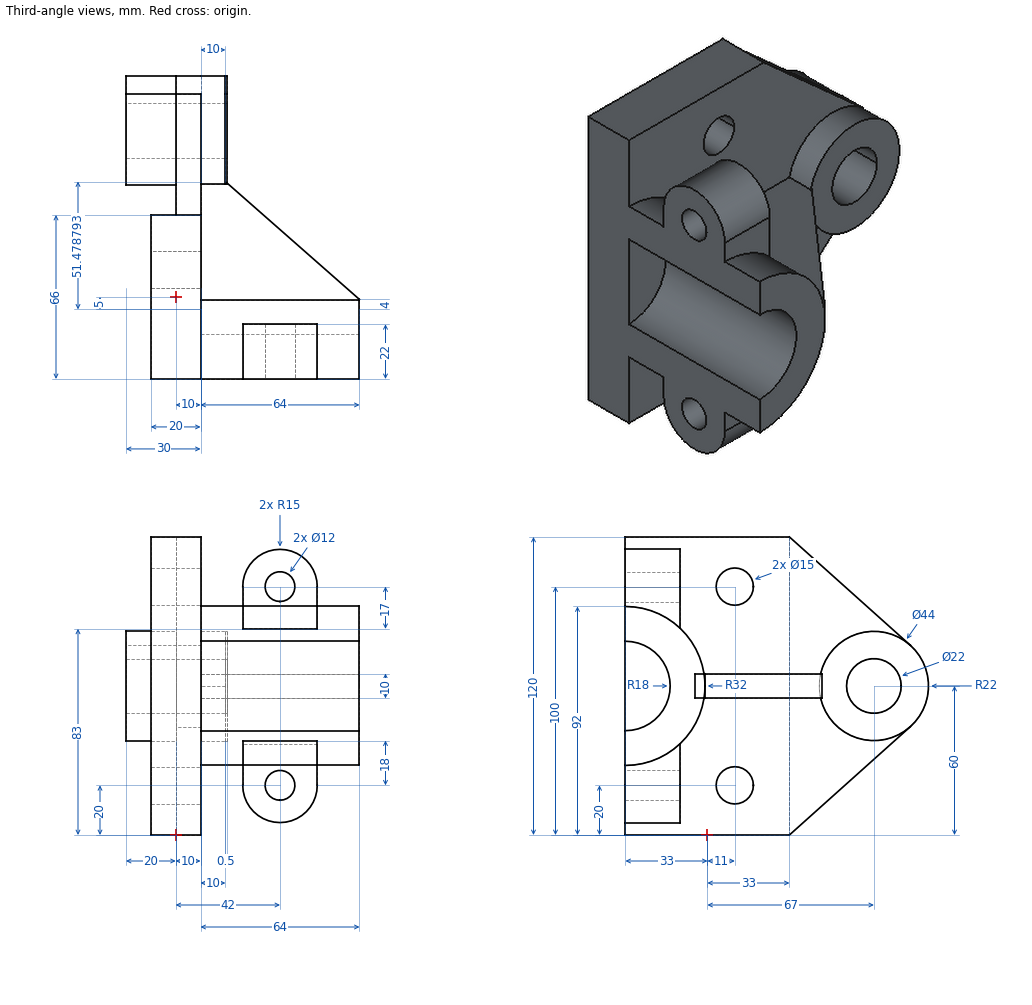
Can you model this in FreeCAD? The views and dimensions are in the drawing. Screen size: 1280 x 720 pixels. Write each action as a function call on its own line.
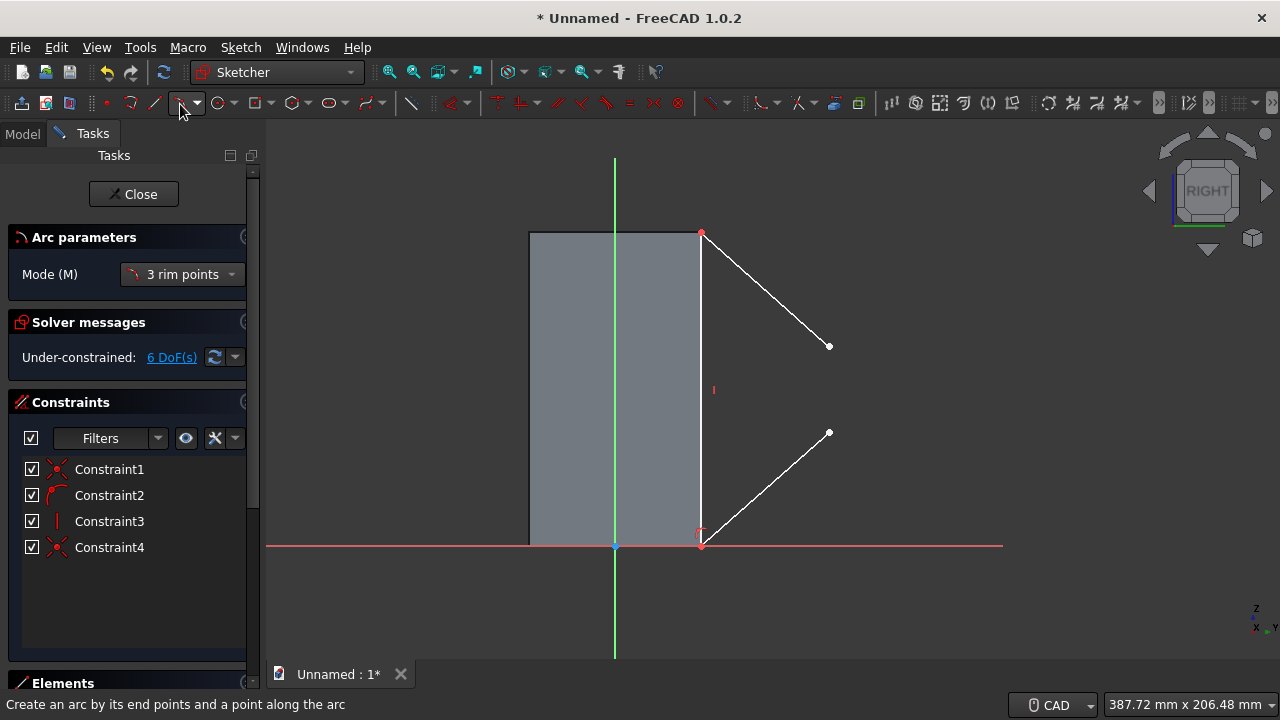
click(829, 433)
click(829, 347)
click(848, 389)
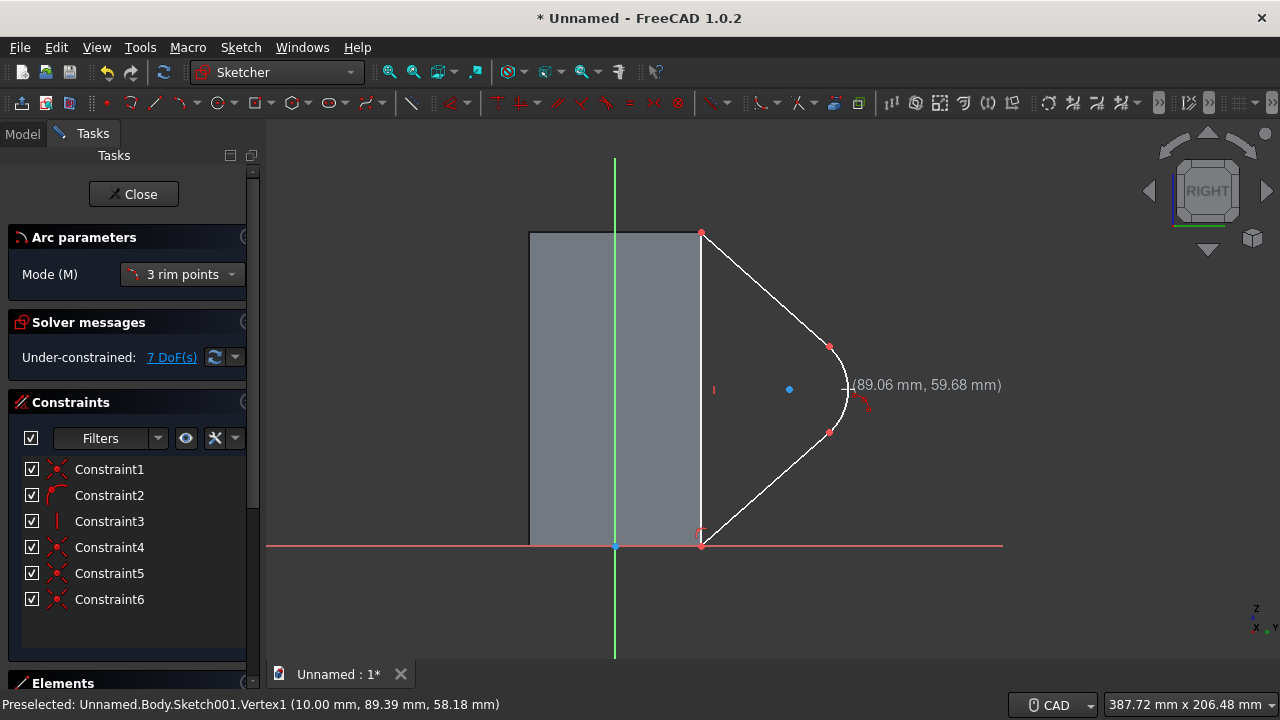
click(218, 104)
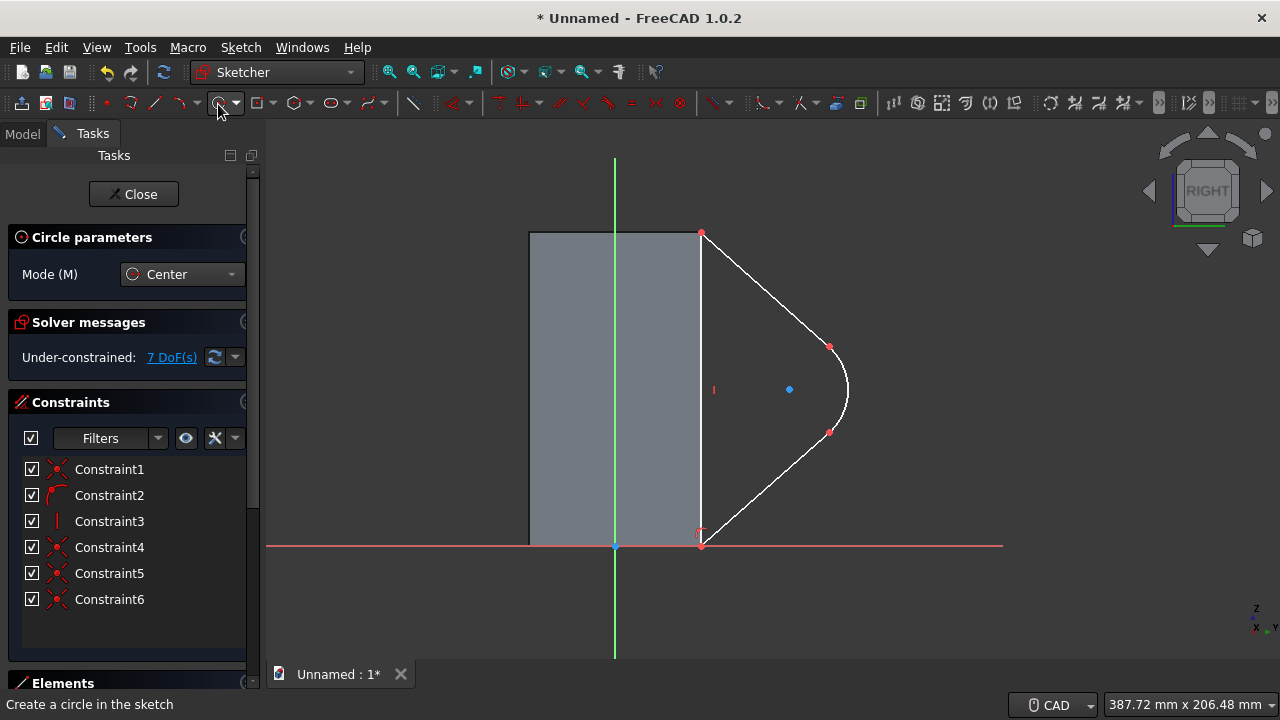
click(790, 389)
click(811, 369)
key(Escape)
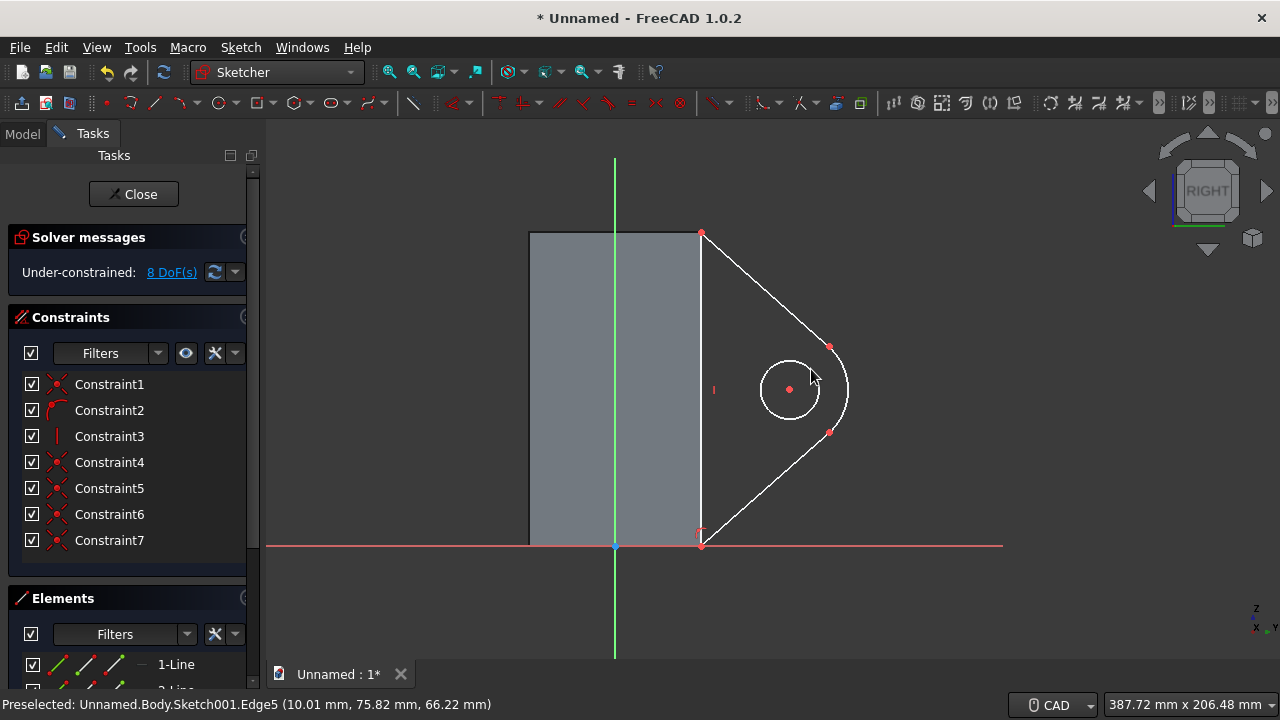
click(791, 313)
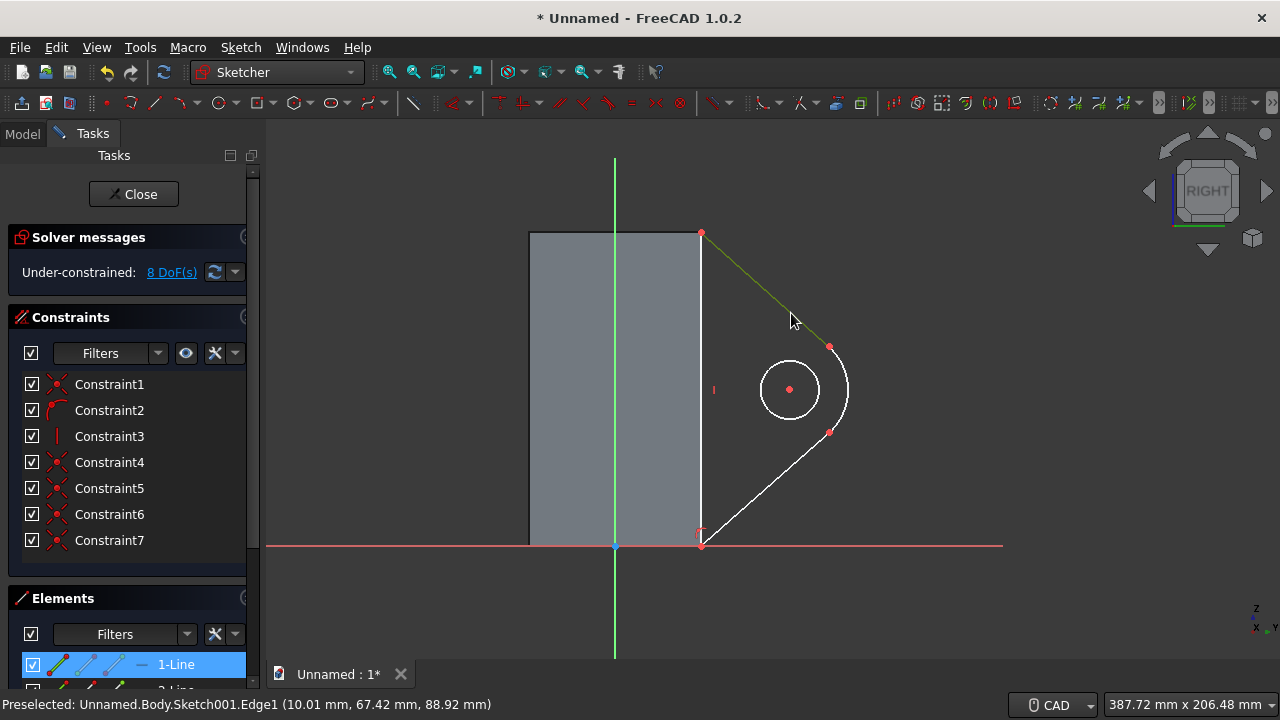
click(845, 409)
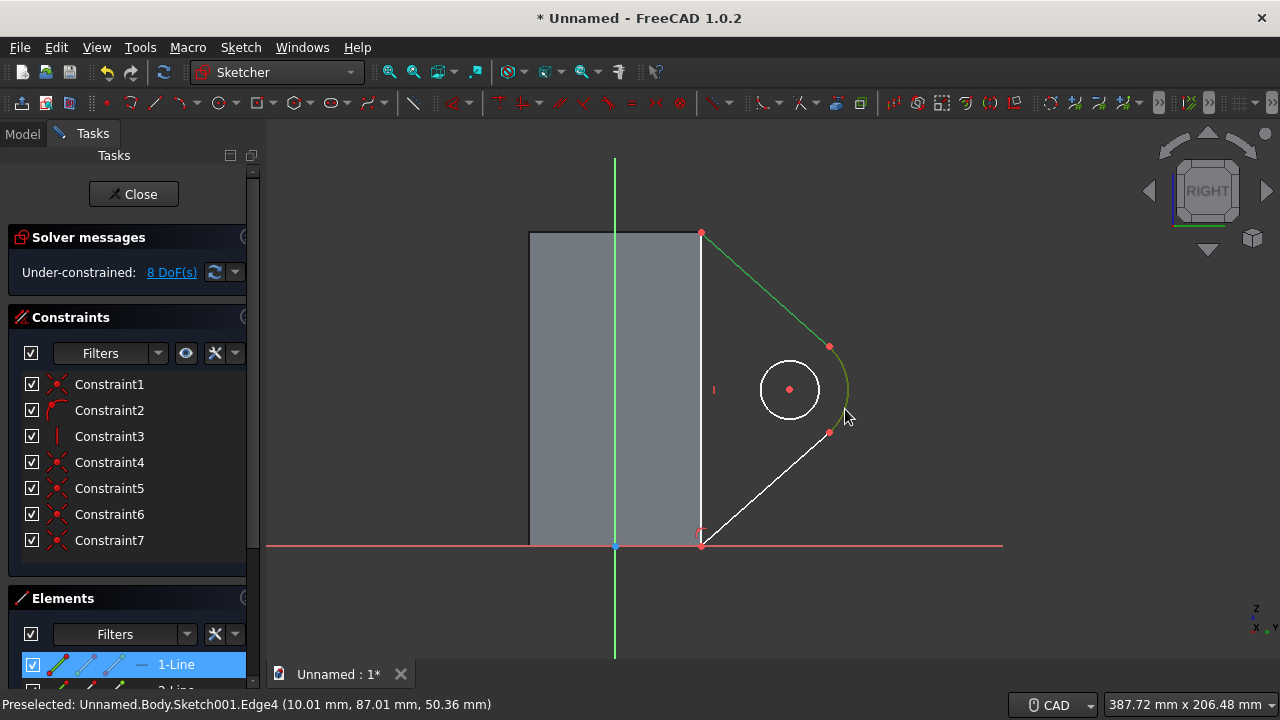
click(608, 104)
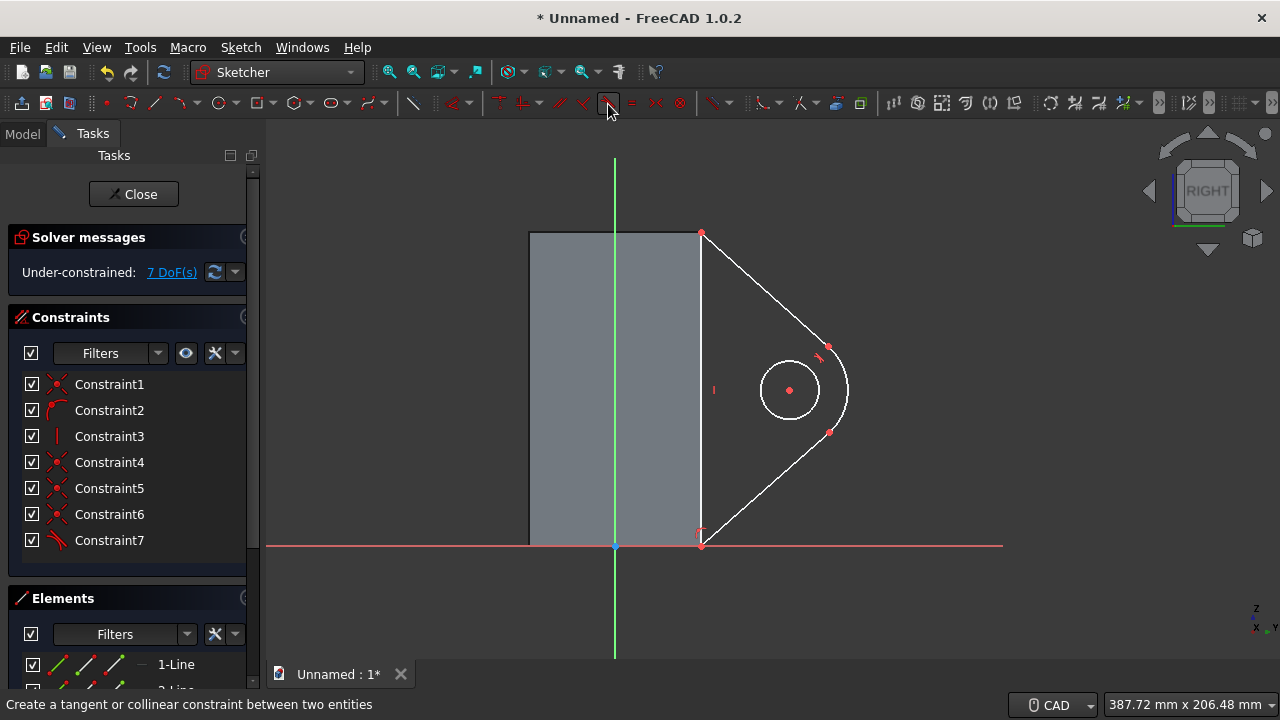
click(739, 512)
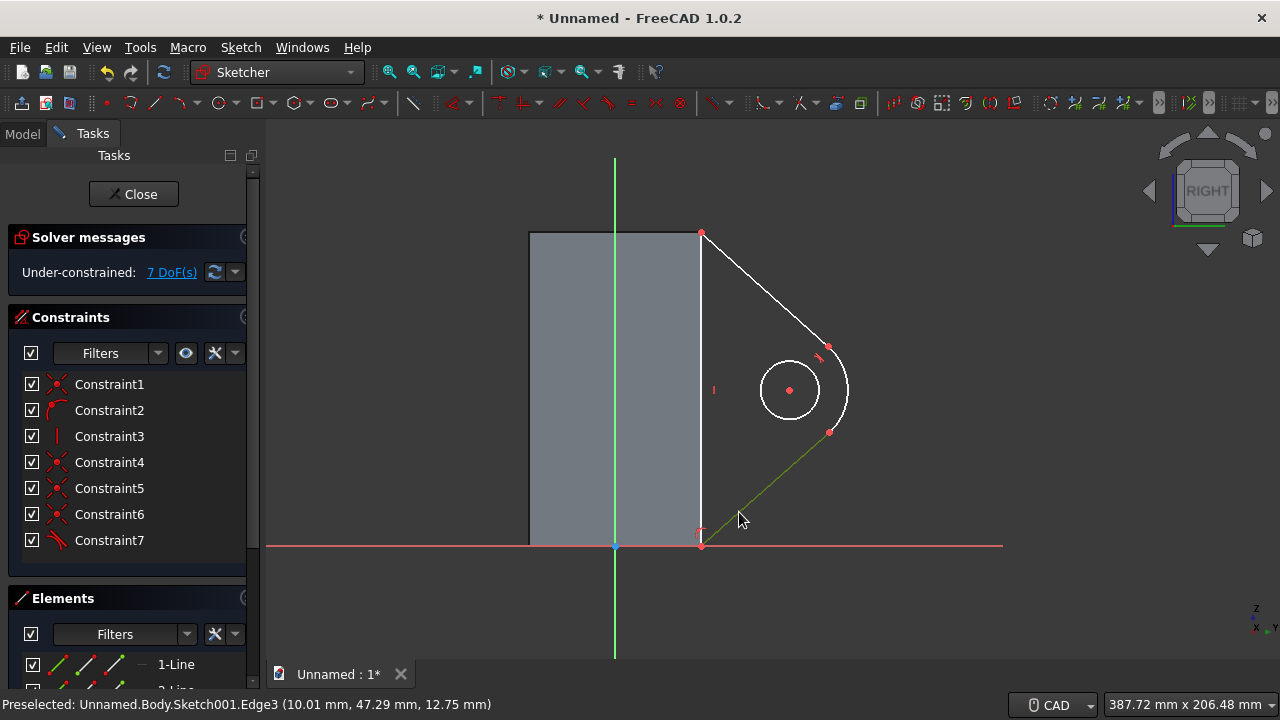
click(845, 409)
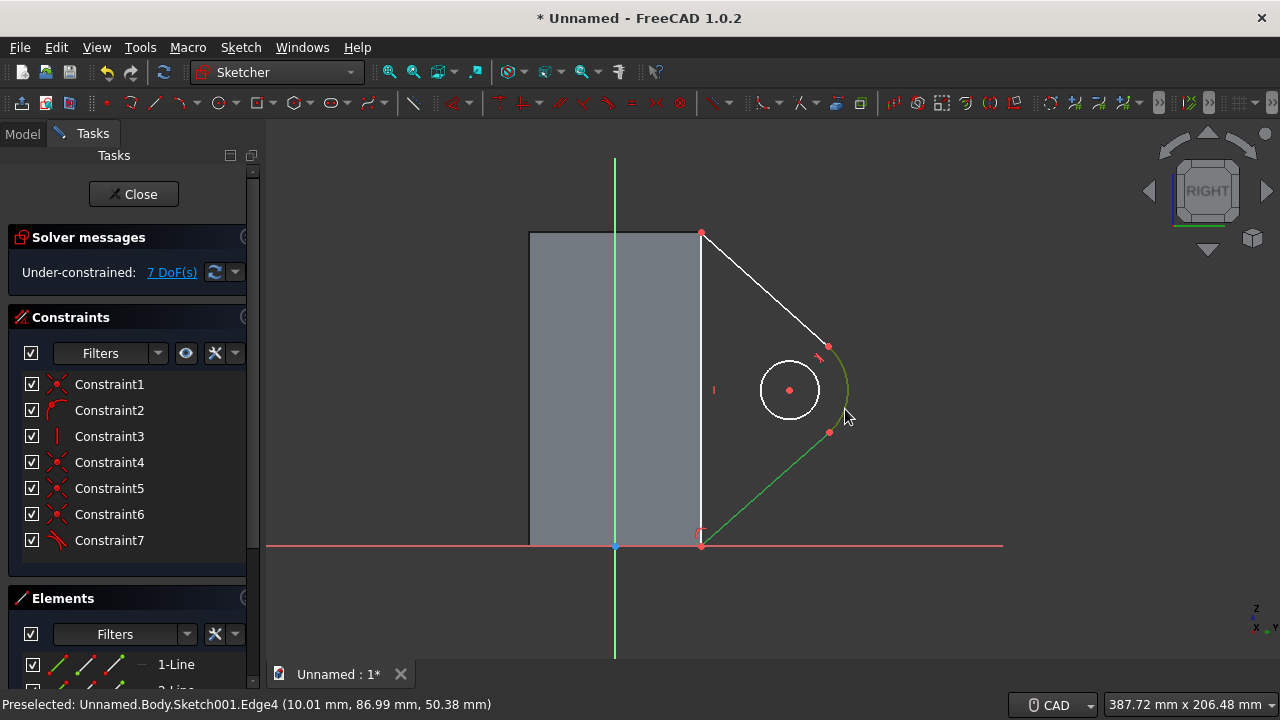
click(608, 104)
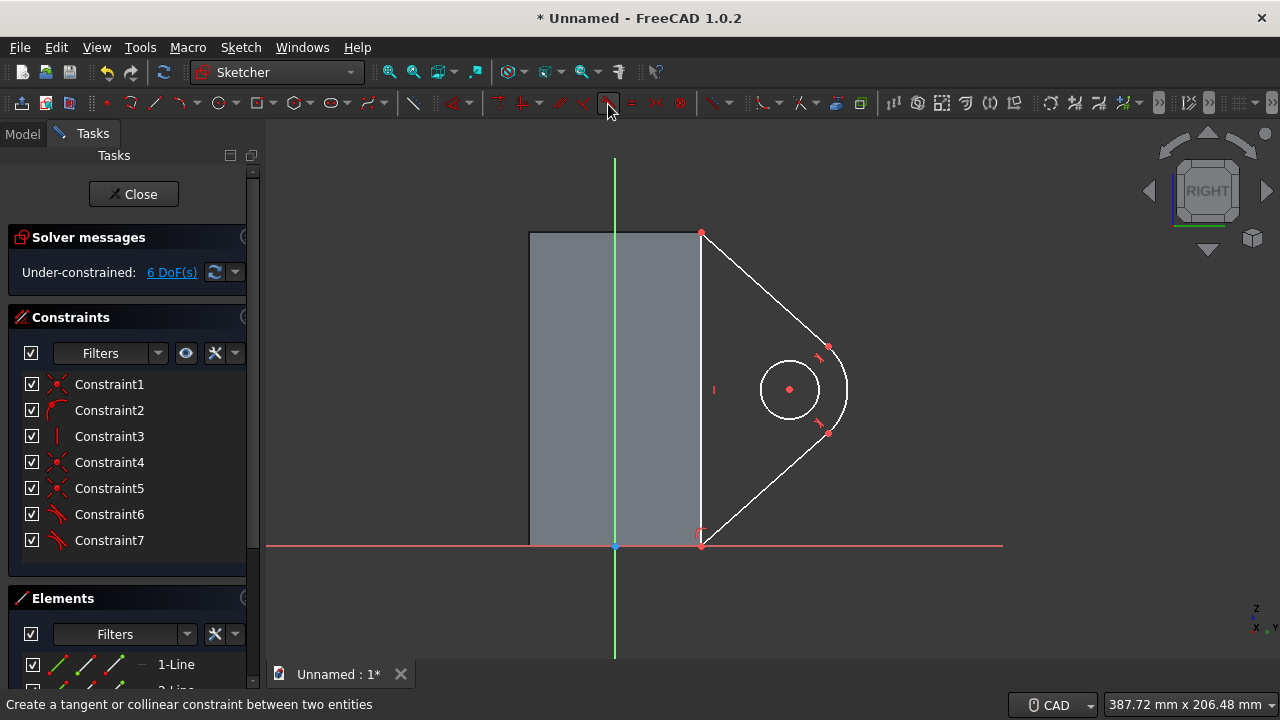
click(452, 104)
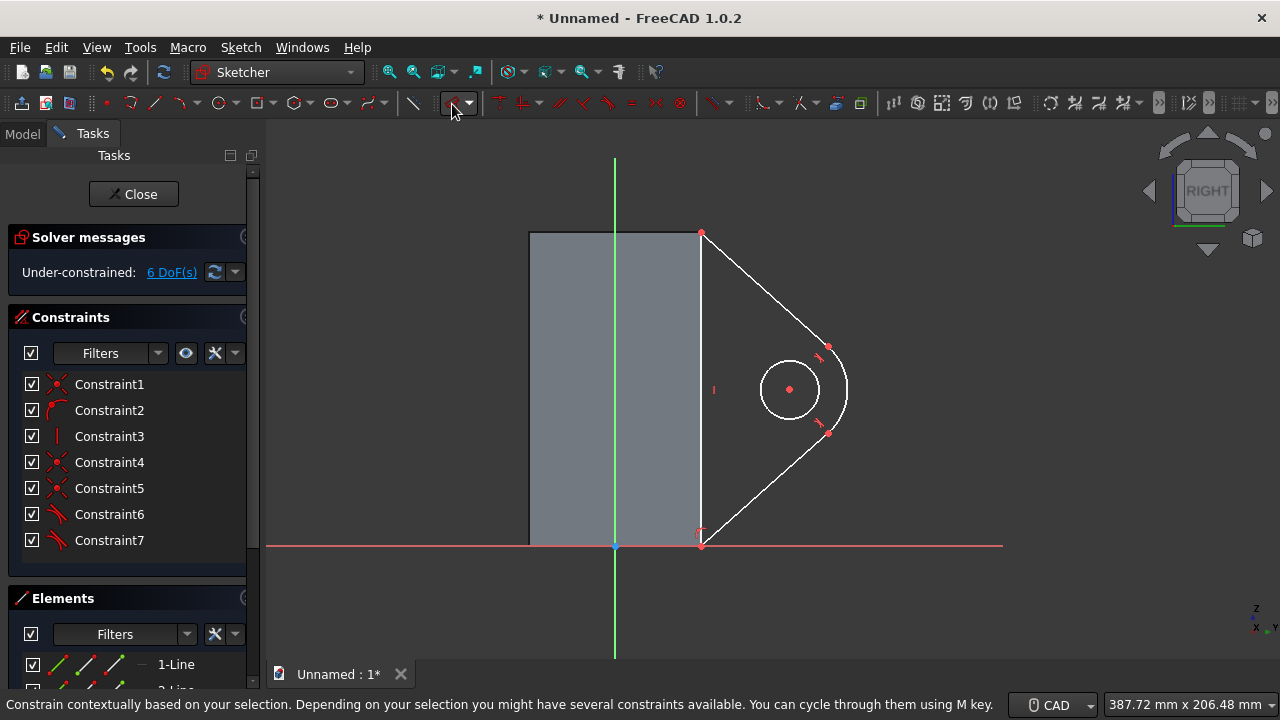
click(844, 409)
click(874, 420)